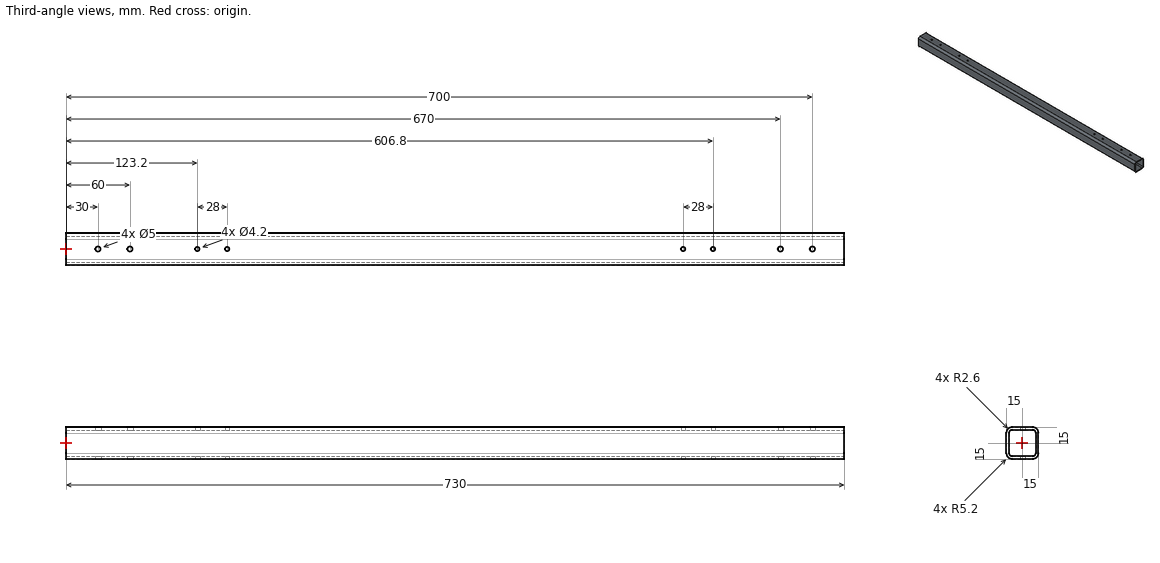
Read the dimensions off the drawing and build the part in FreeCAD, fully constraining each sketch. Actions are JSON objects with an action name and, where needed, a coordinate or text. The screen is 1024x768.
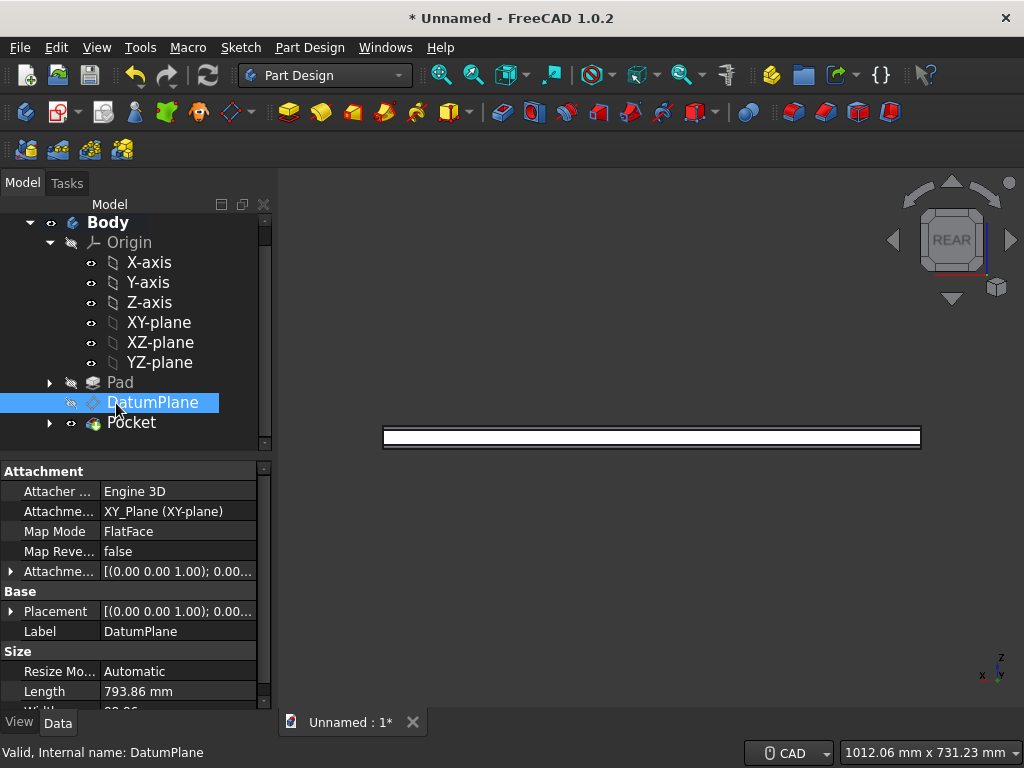
{"action": "key", "text": "0"}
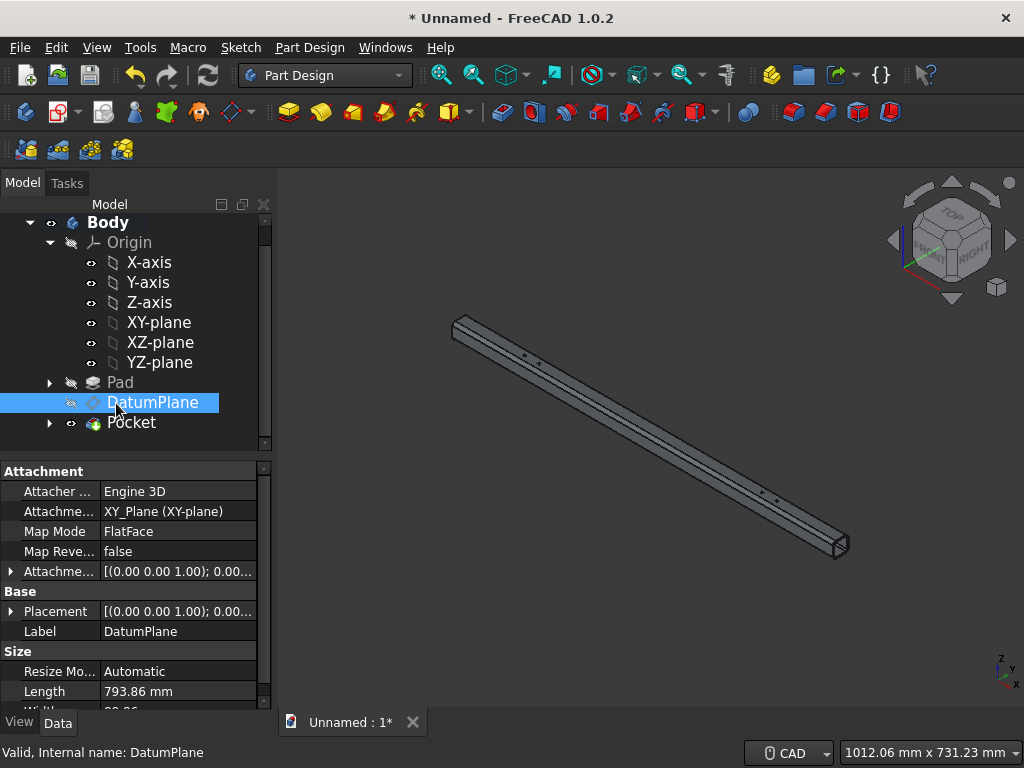
{"action": "key", "text": "2"}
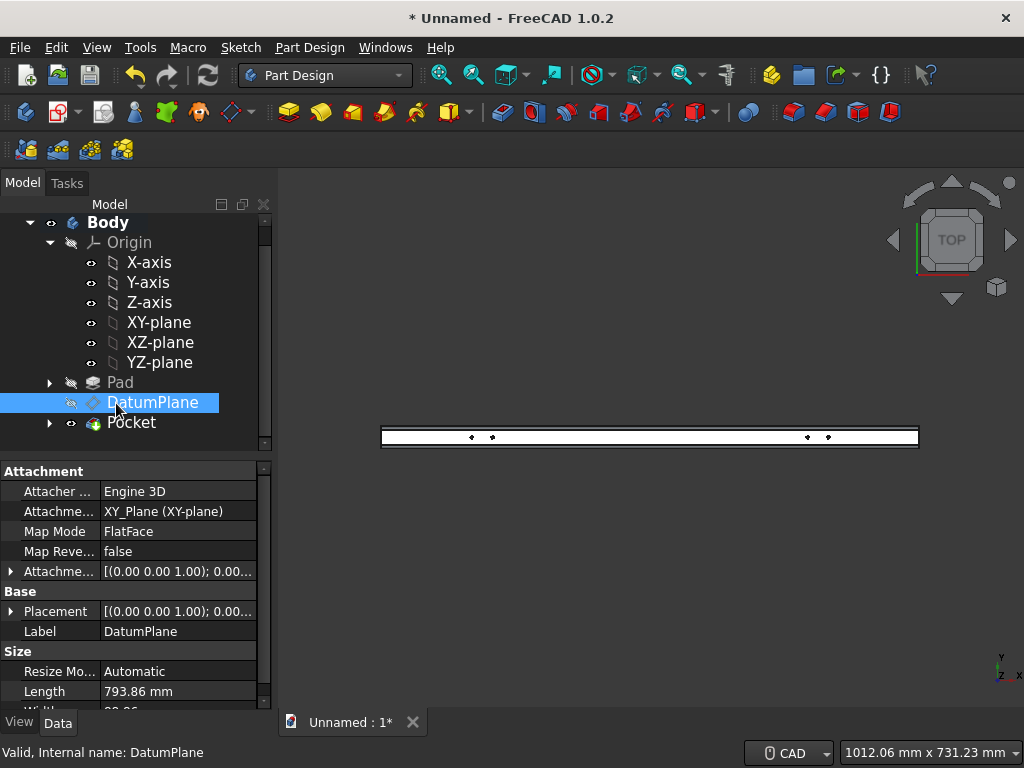
{"action": "key", "text": "4"}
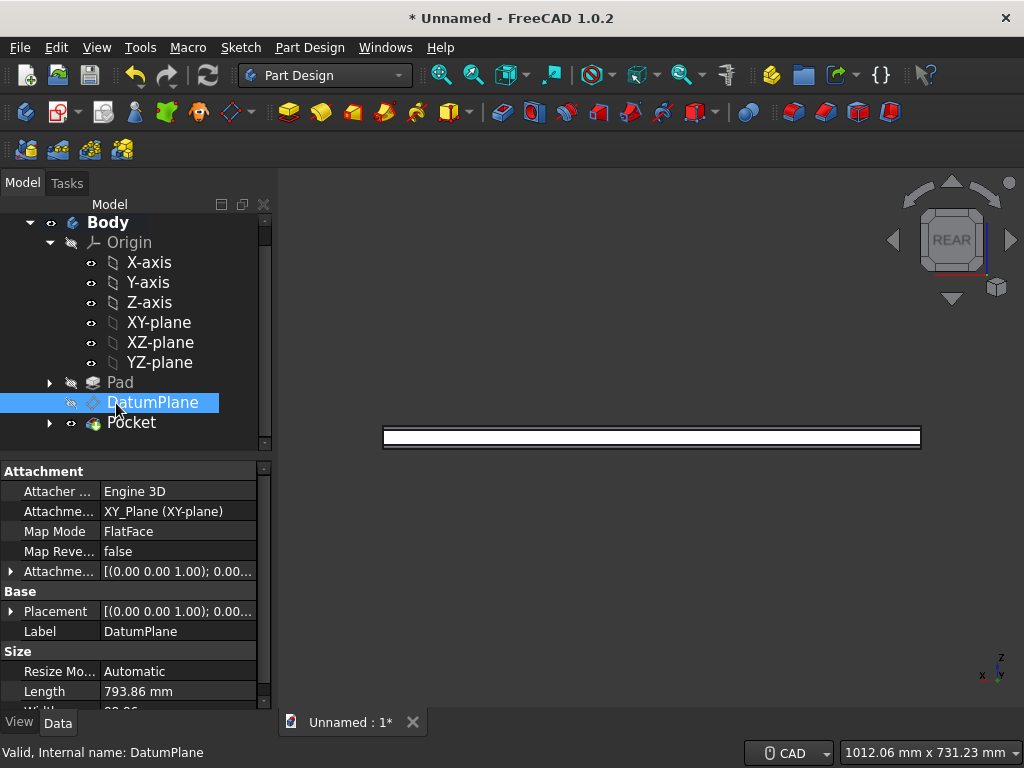
{"action": "left_click", "coordinate": [136, 323]}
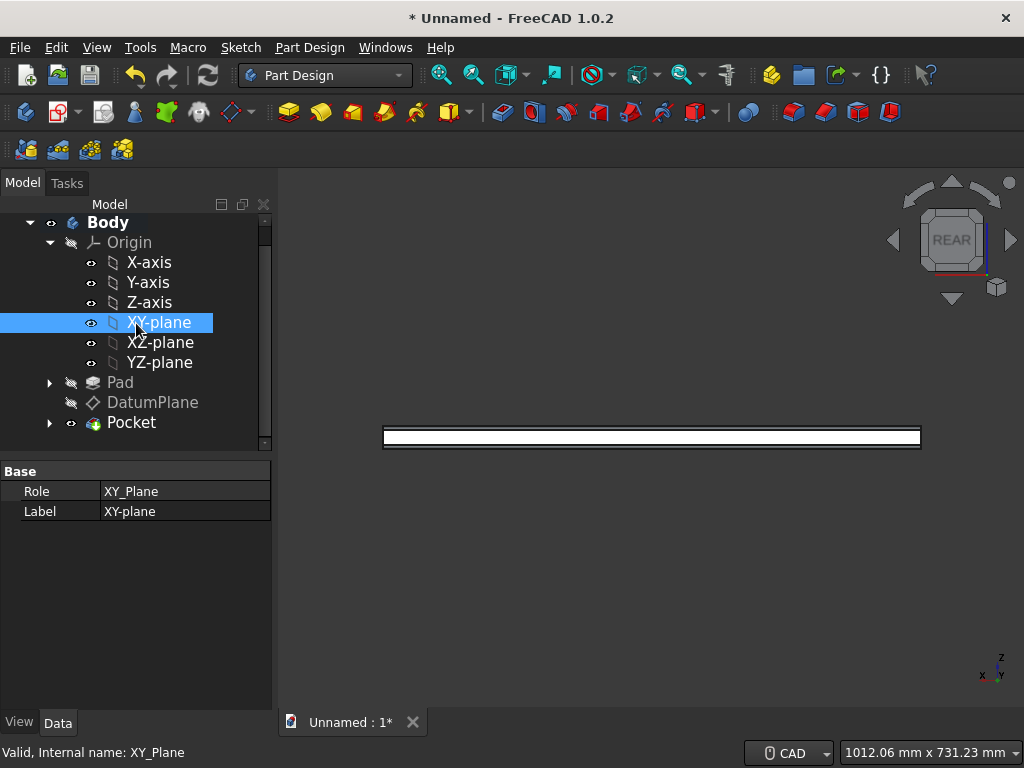
{"action": "left_click", "coordinate": [232, 112]}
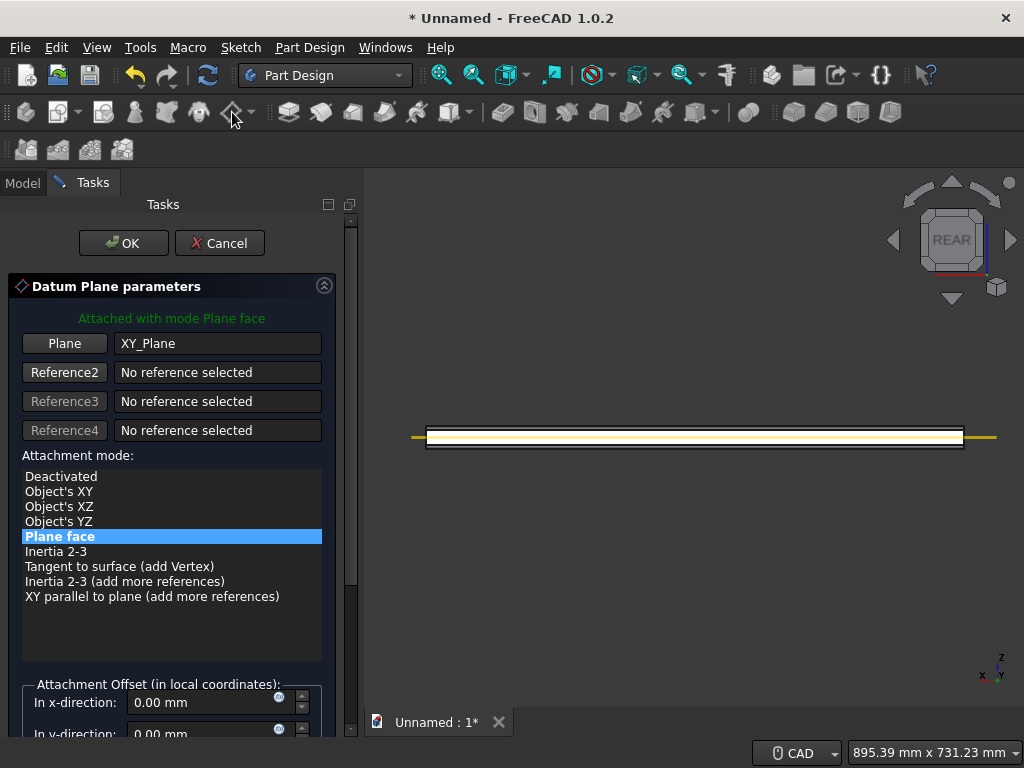
{"action": "scroll", "coordinate": [351, 475], "scroll_direction": "down", "scroll_amount": 2}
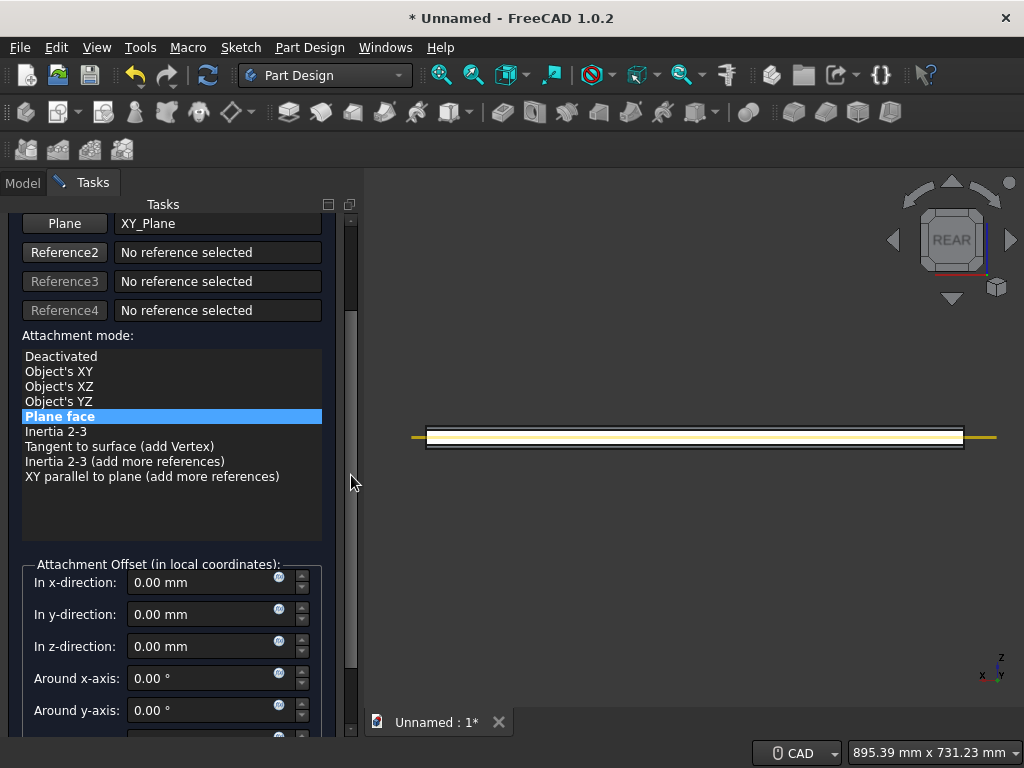
{"action": "triple_click", "coordinate": [210, 646]}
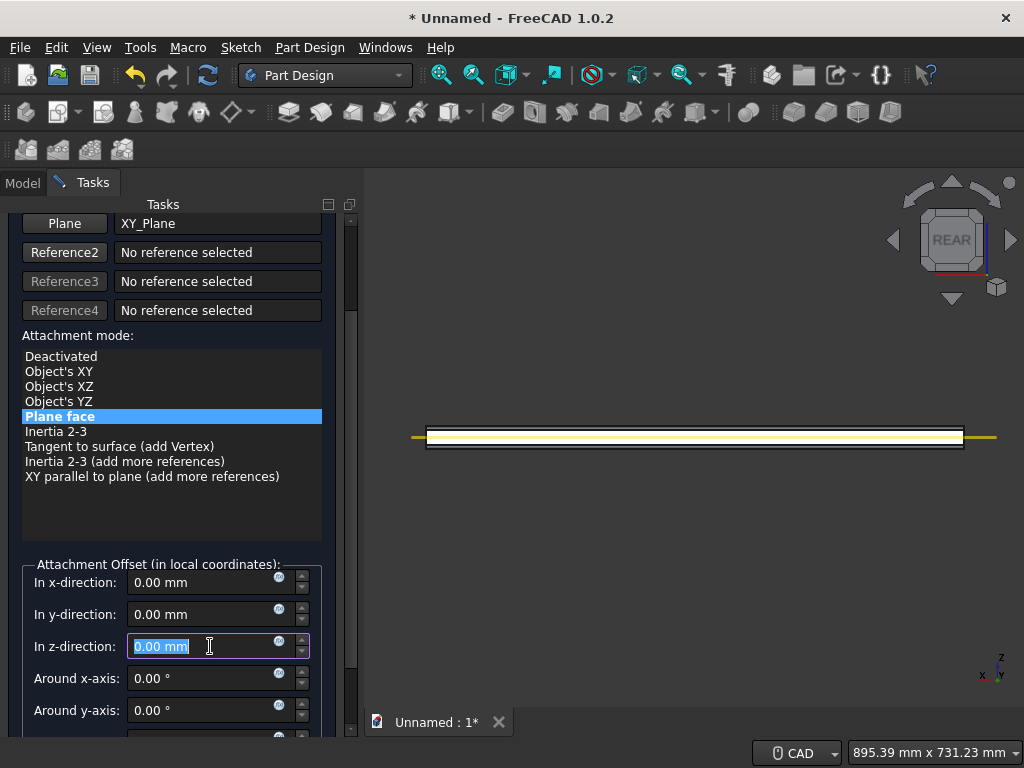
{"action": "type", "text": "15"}
{"action": "key", "text": "Tab"}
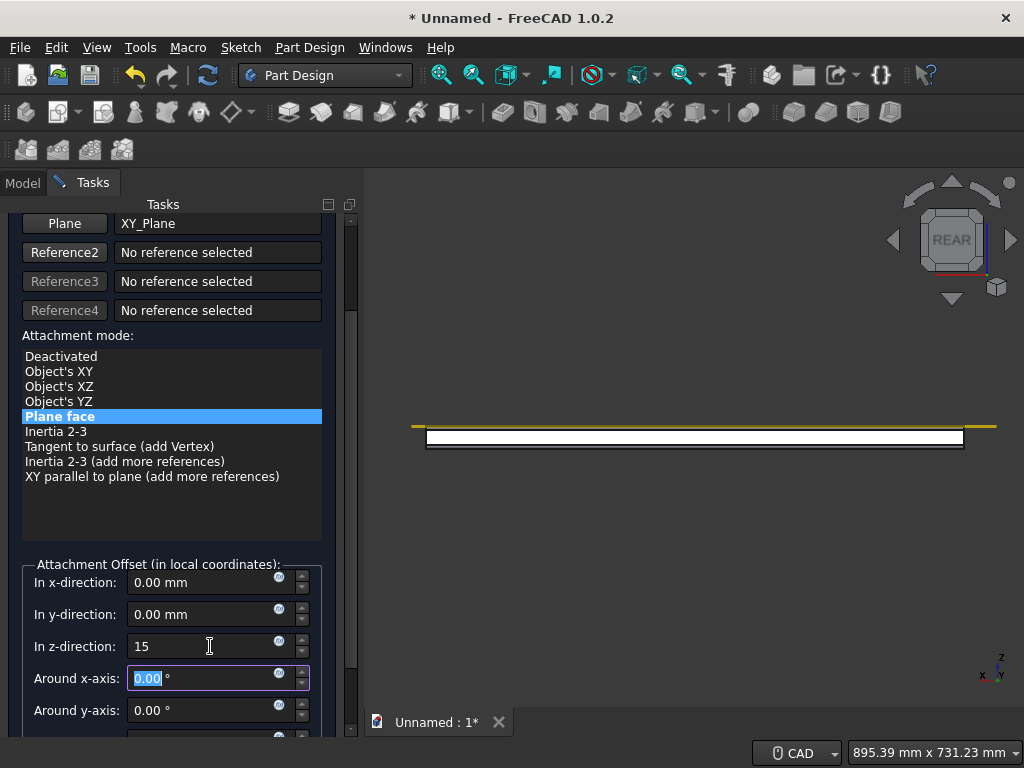
{"action": "scroll", "coordinate": [351, 475], "scroll_direction": "up", "scroll_amount": 3}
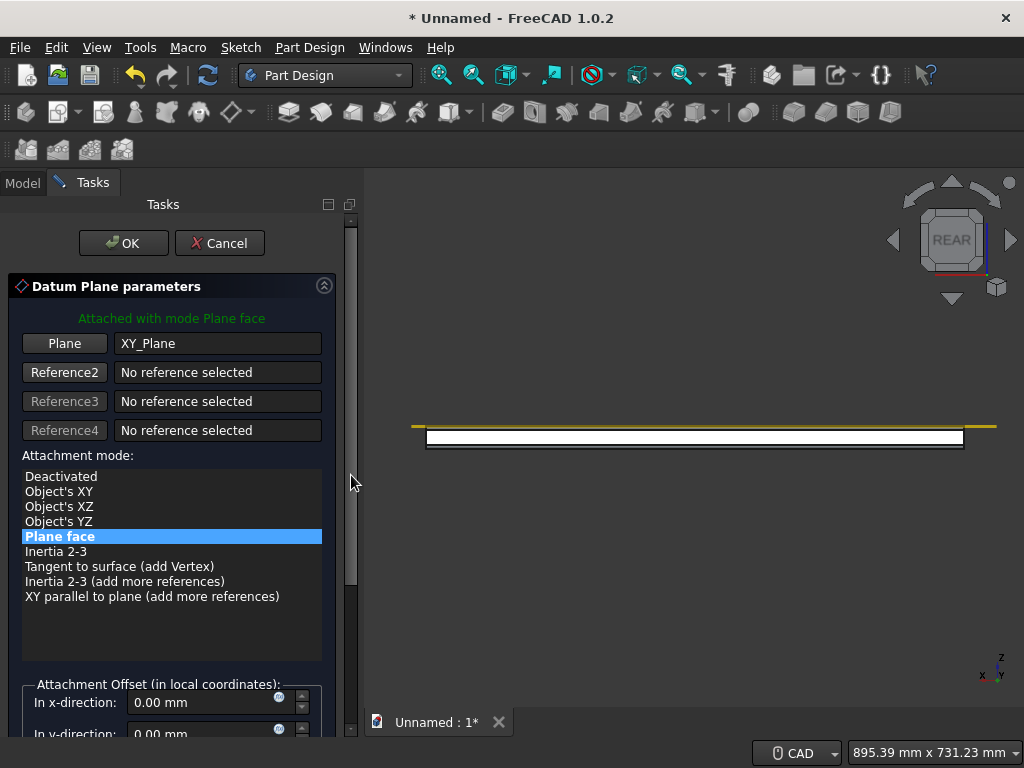
{"action": "left_click", "coordinate": [124, 243]}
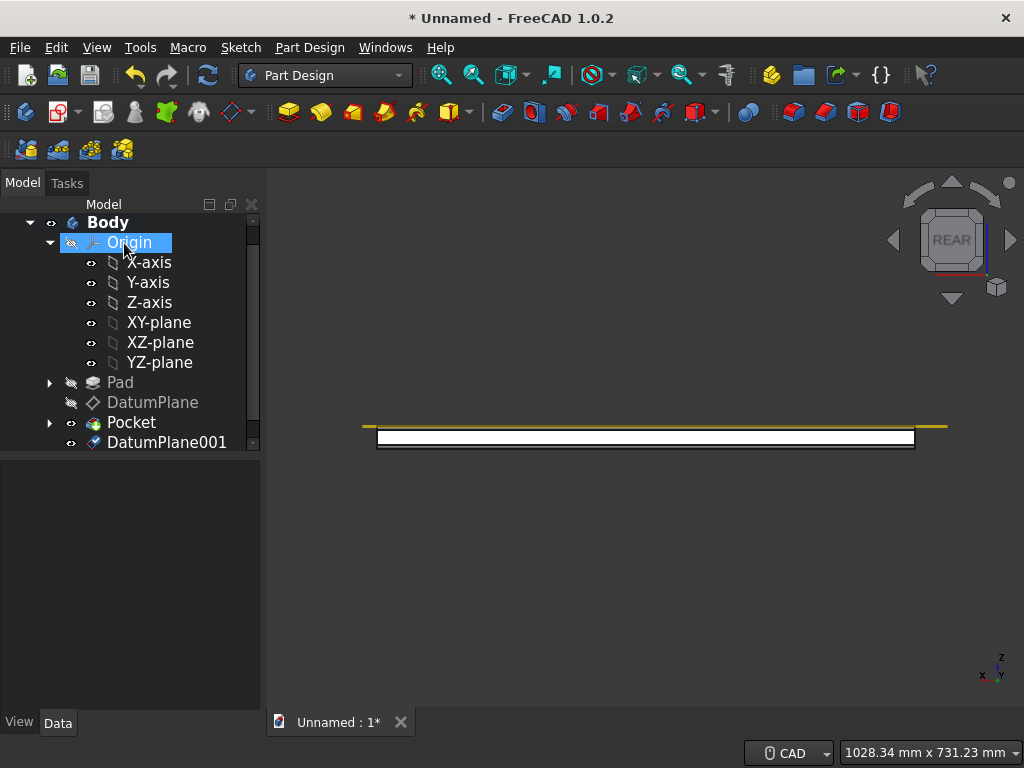
{"action": "left_click", "coordinate": [116, 443]}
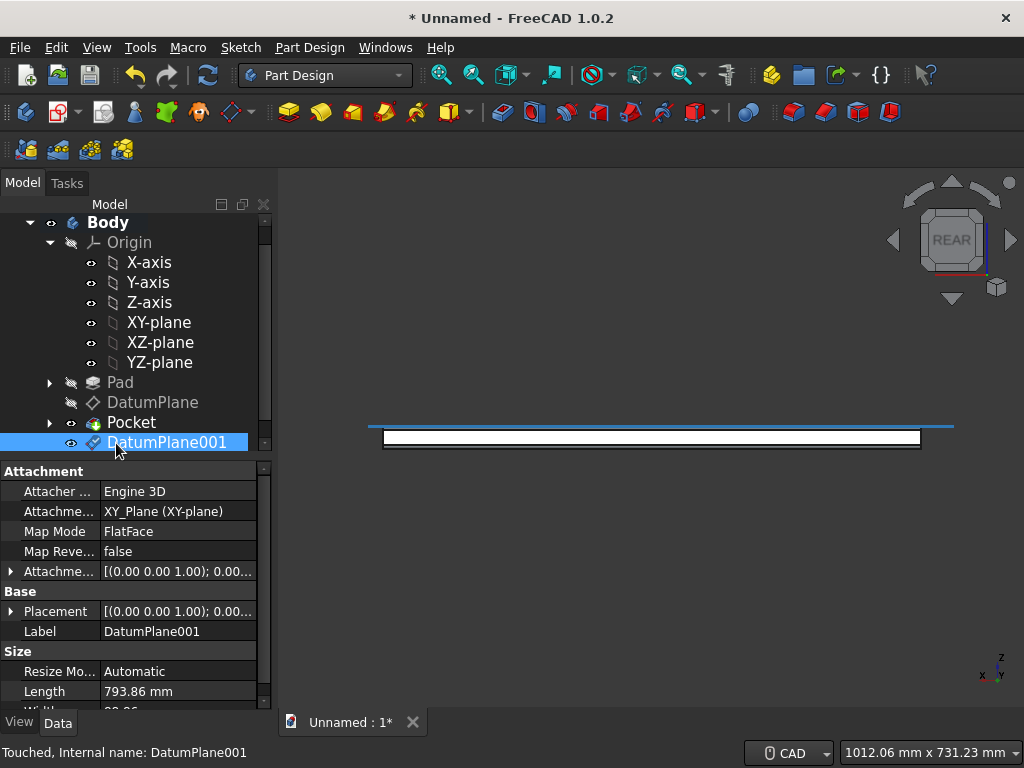
{"action": "left_click", "coordinate": [58, 112]}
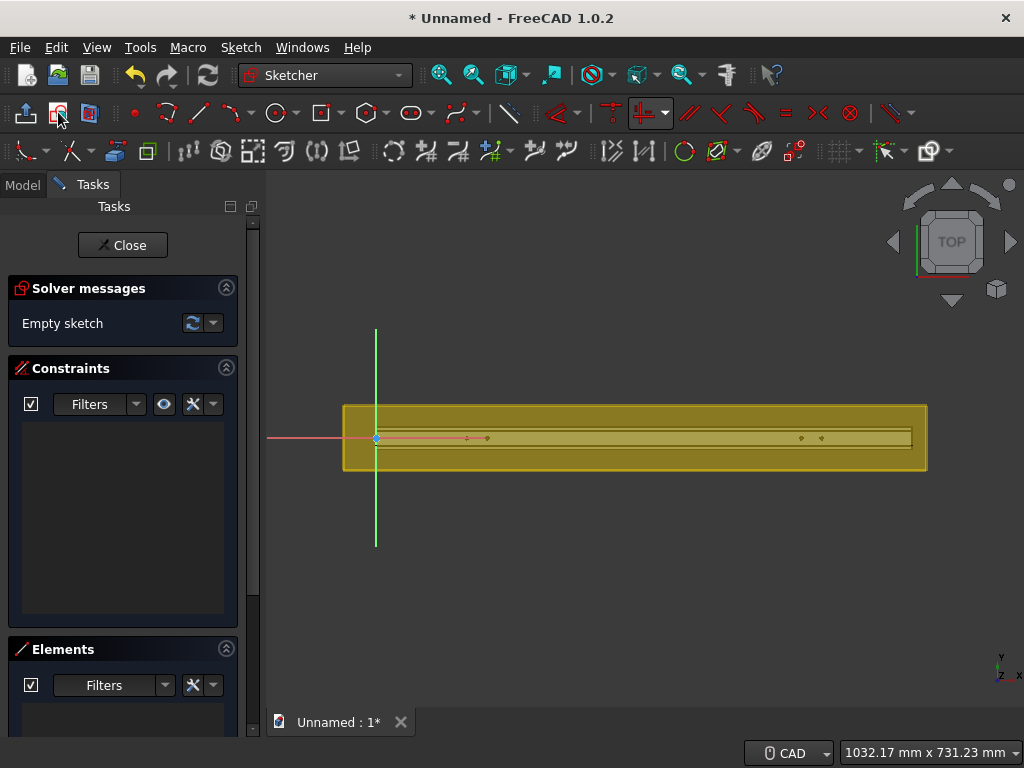
{"action": "scroll", "coordinate": [317, 439], "scroll_direction": "down", "scroll_amount": 1}